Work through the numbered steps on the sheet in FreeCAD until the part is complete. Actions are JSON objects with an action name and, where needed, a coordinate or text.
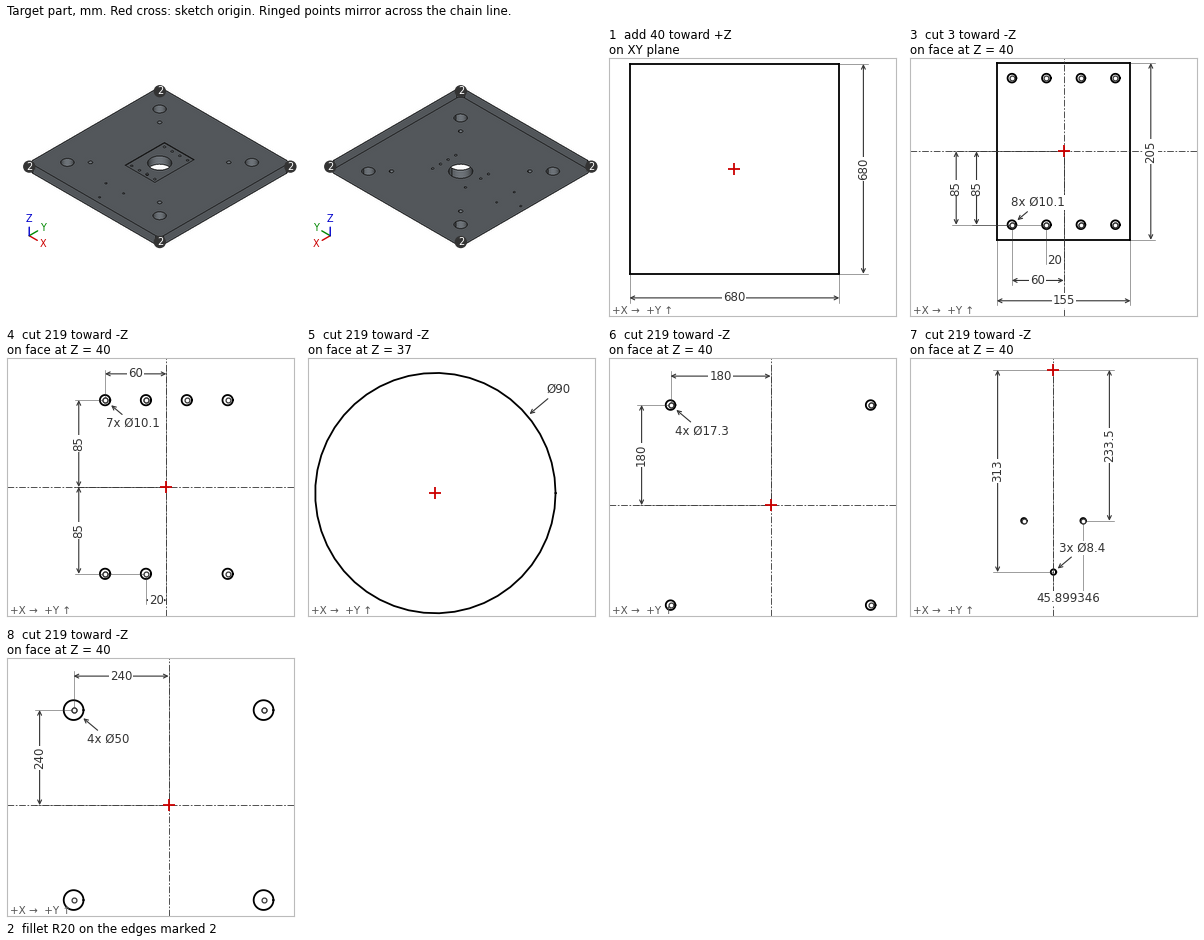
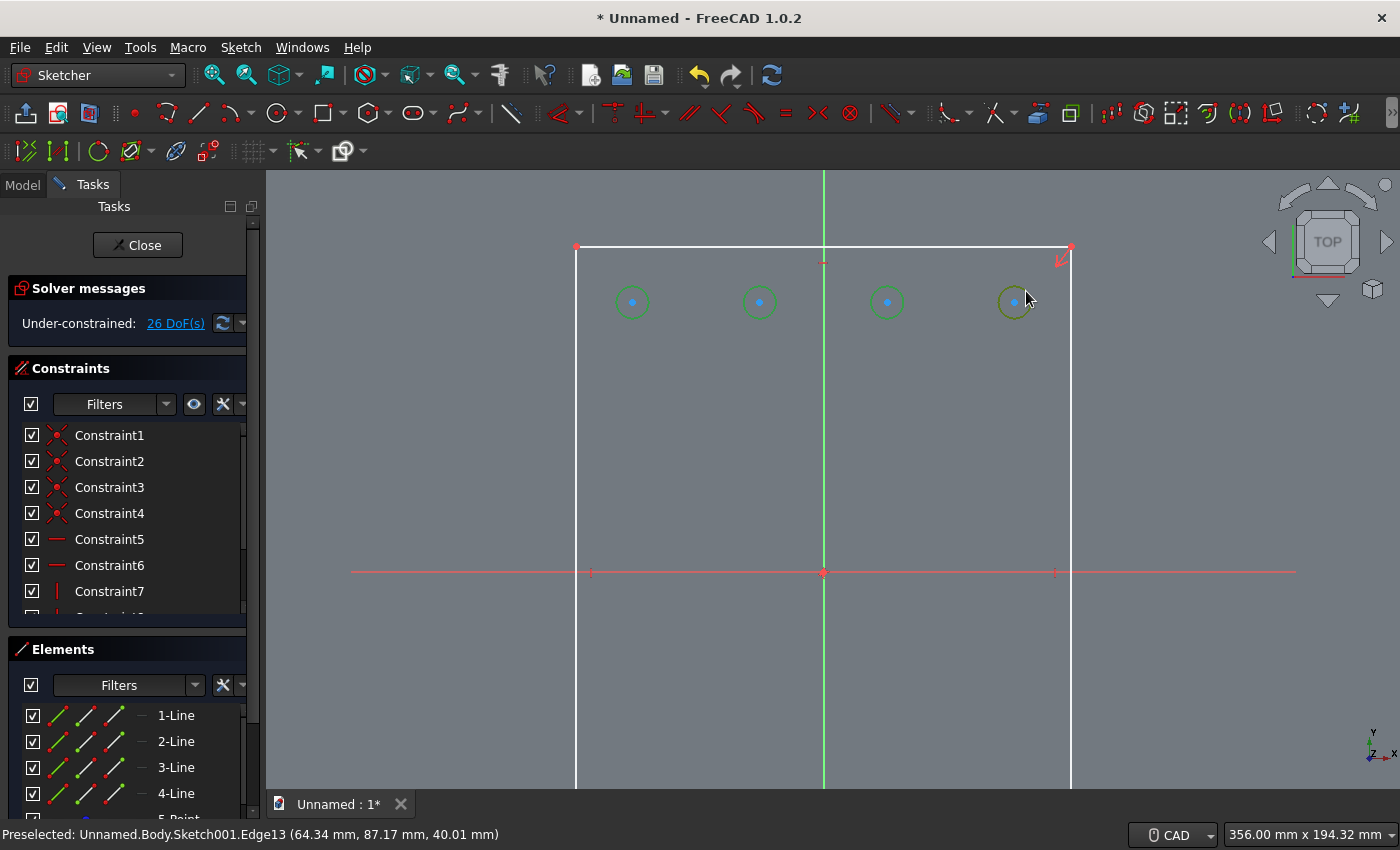
{"action": "left_click", "coordinate": [786, 114]}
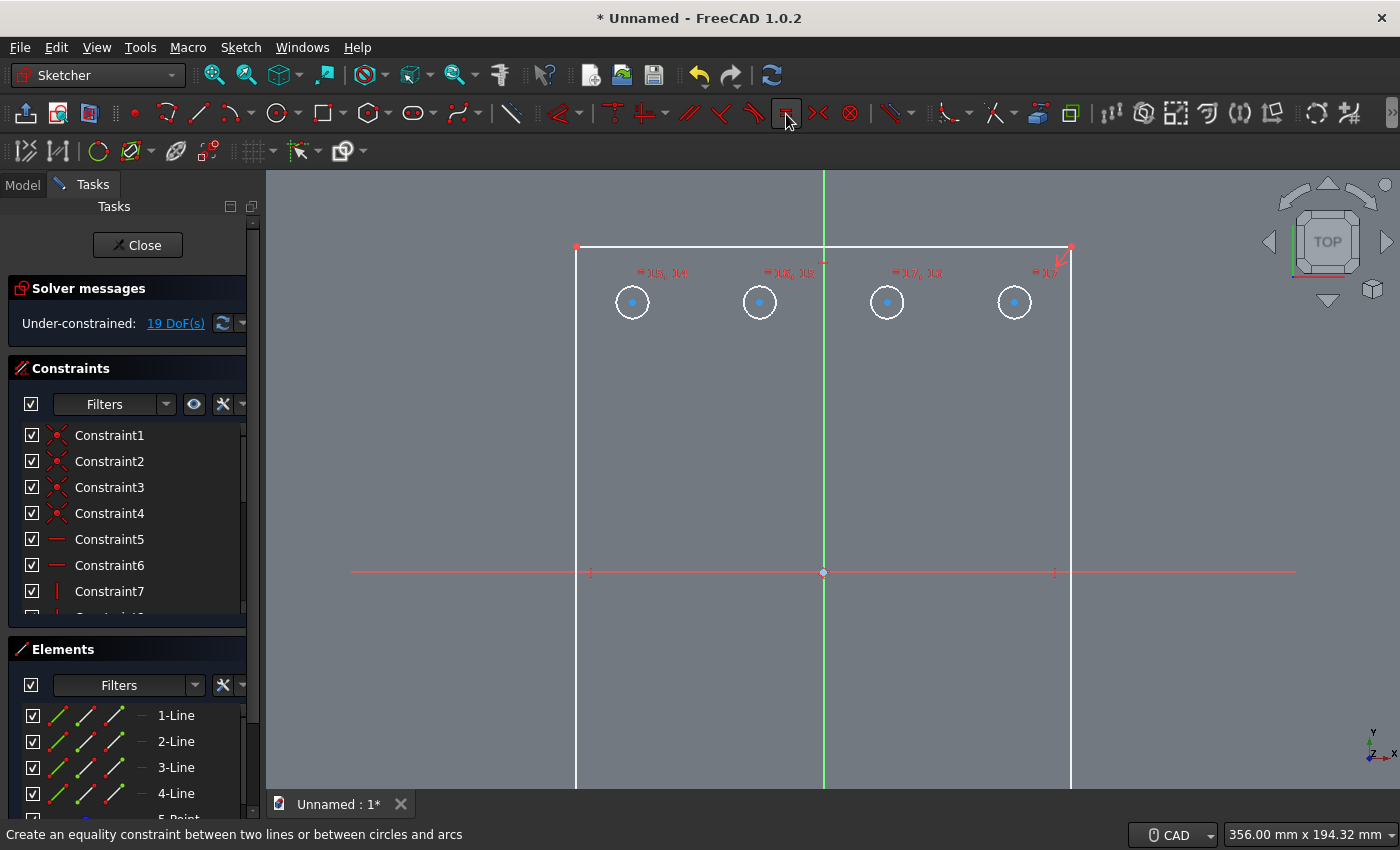
{"action": "scroll", "coordinate": [644, 291], "scroll_direction": "down", "scroll_amount": 2}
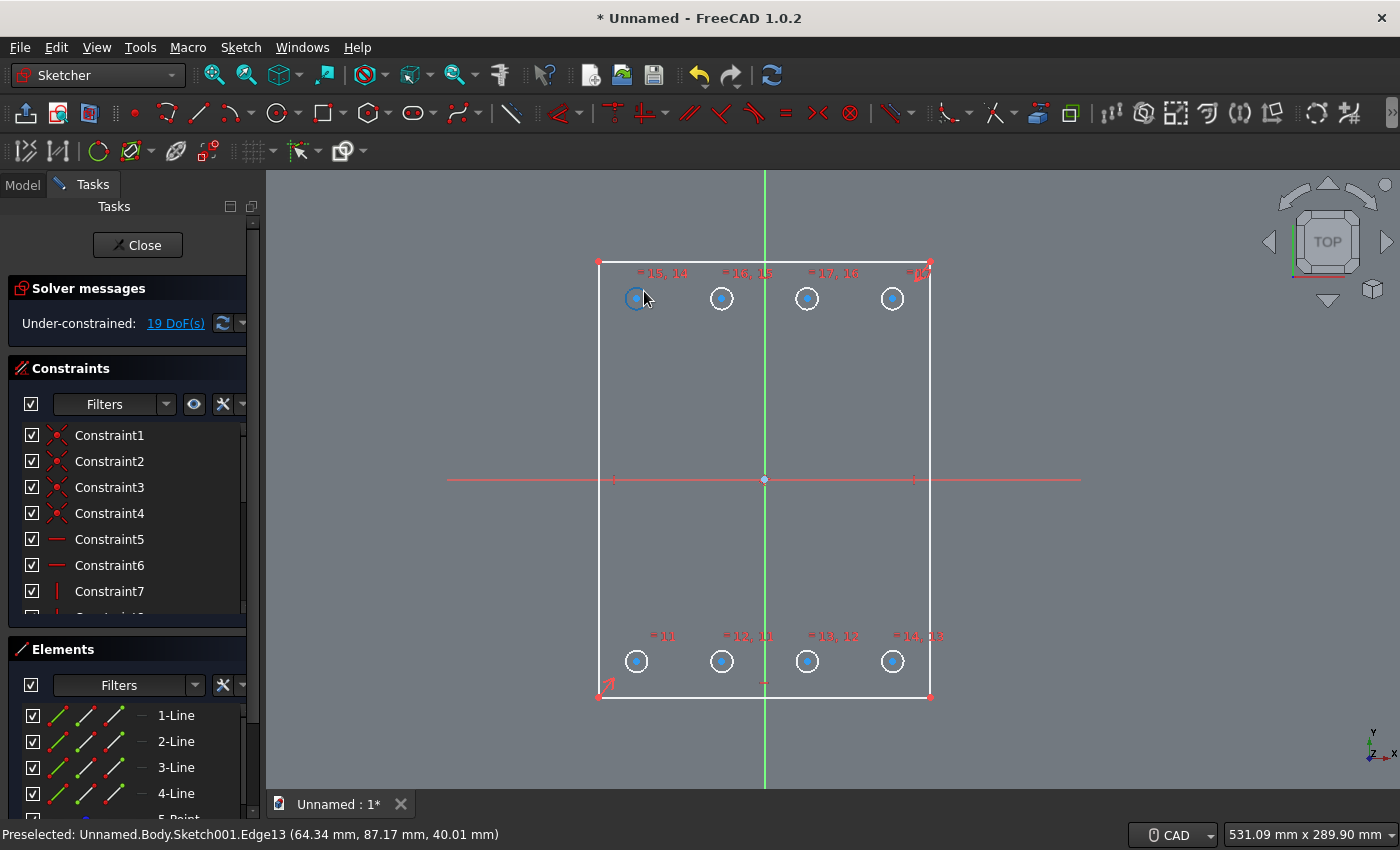
{"action": "left_click", "coordinate": [722, 662]}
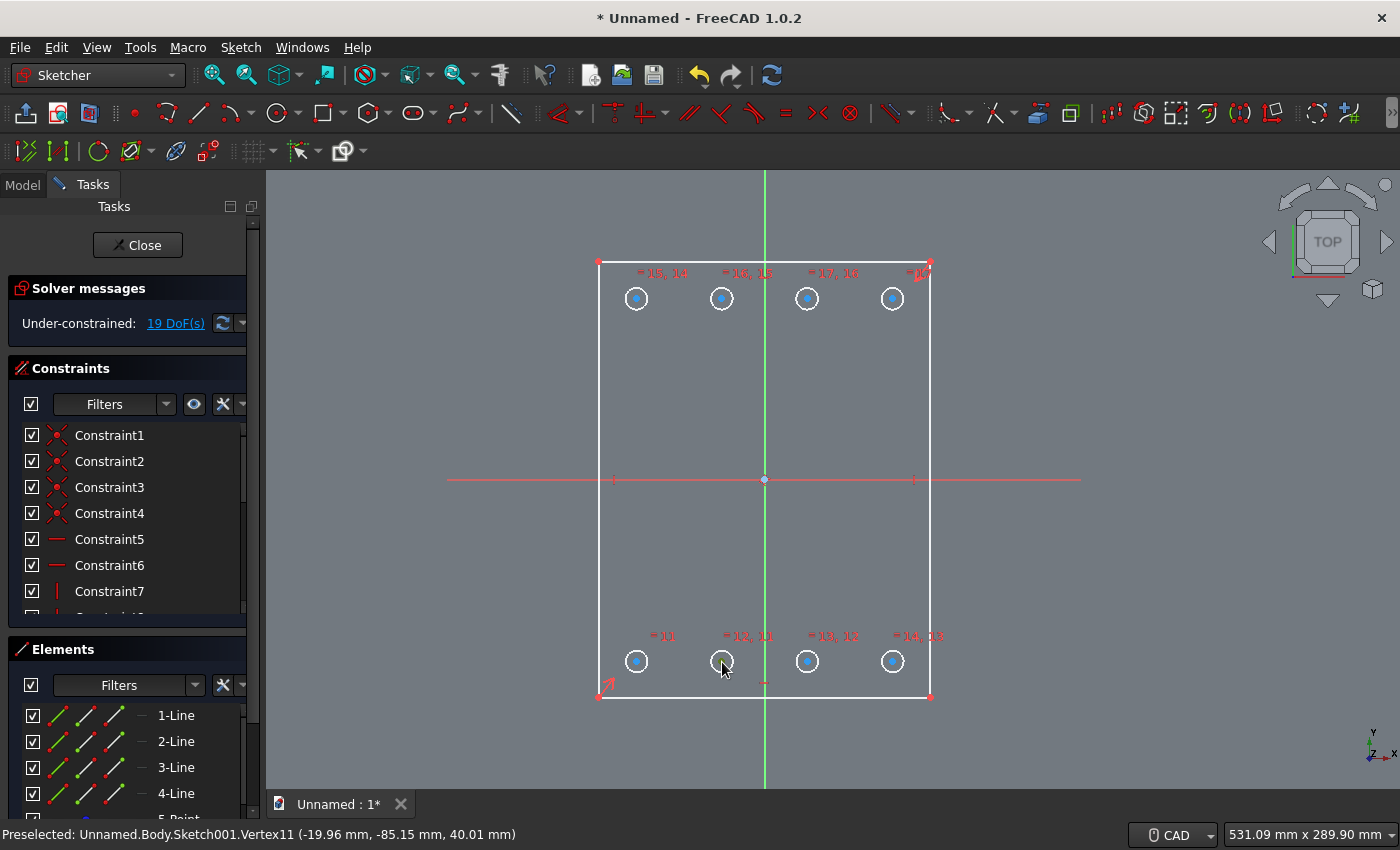
{"action": "left_click", "coordinate": [807, 662]}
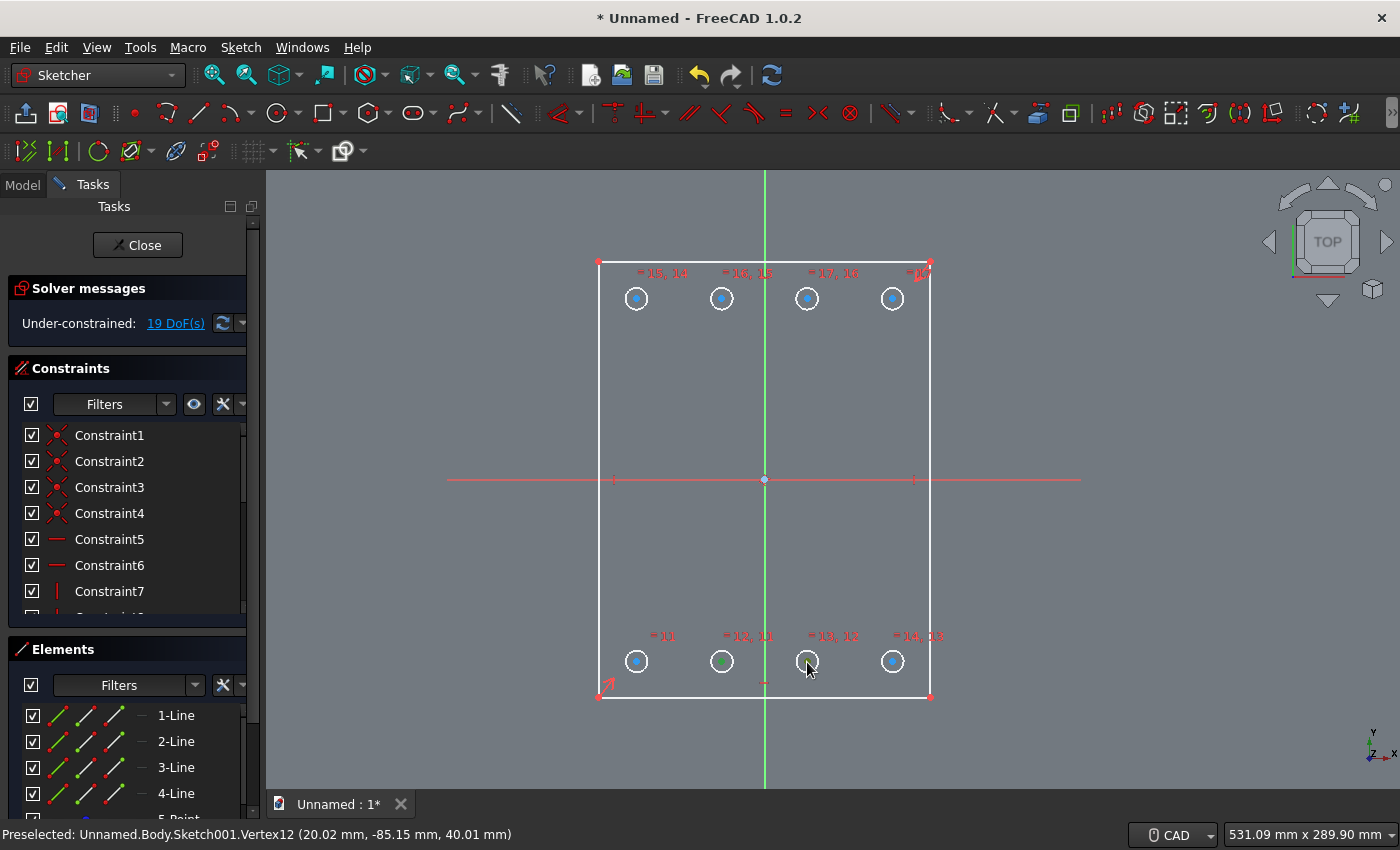
{"action": "left_click", "coordinate": [765, 600]}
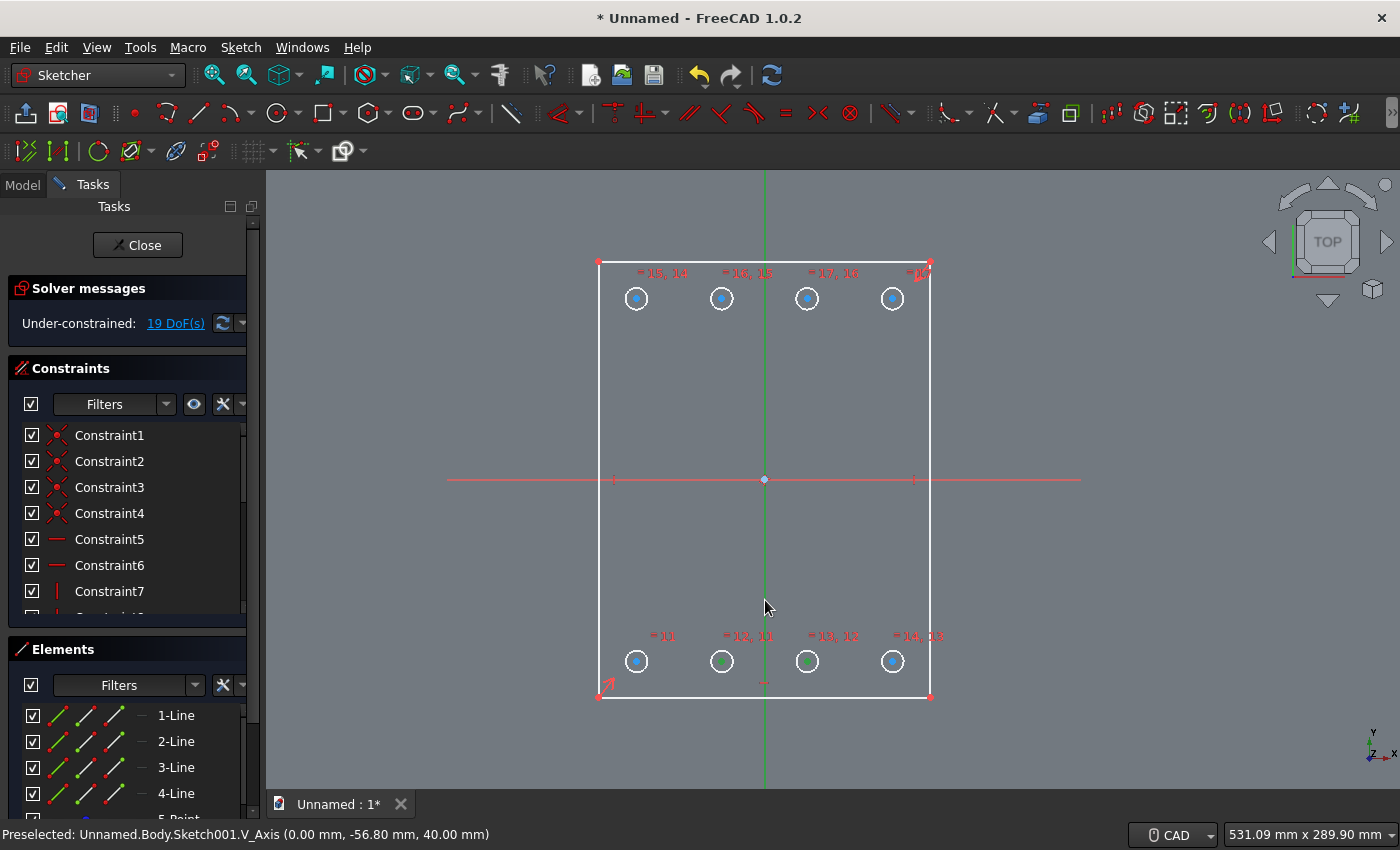
{"action": "left_click", "coordinate": [818, 114]}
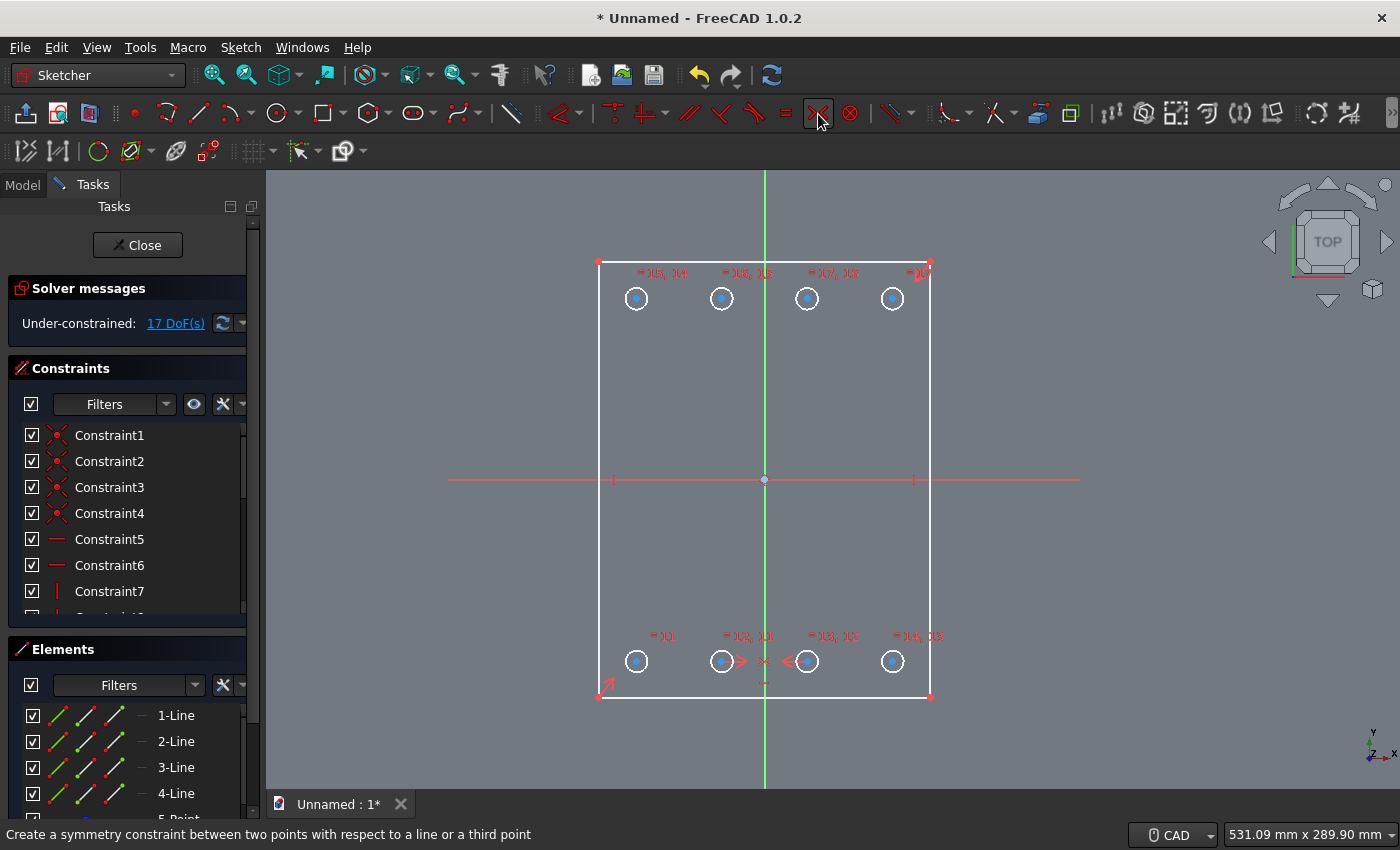
{"action": "left_click", "coordinate": [637, 662]}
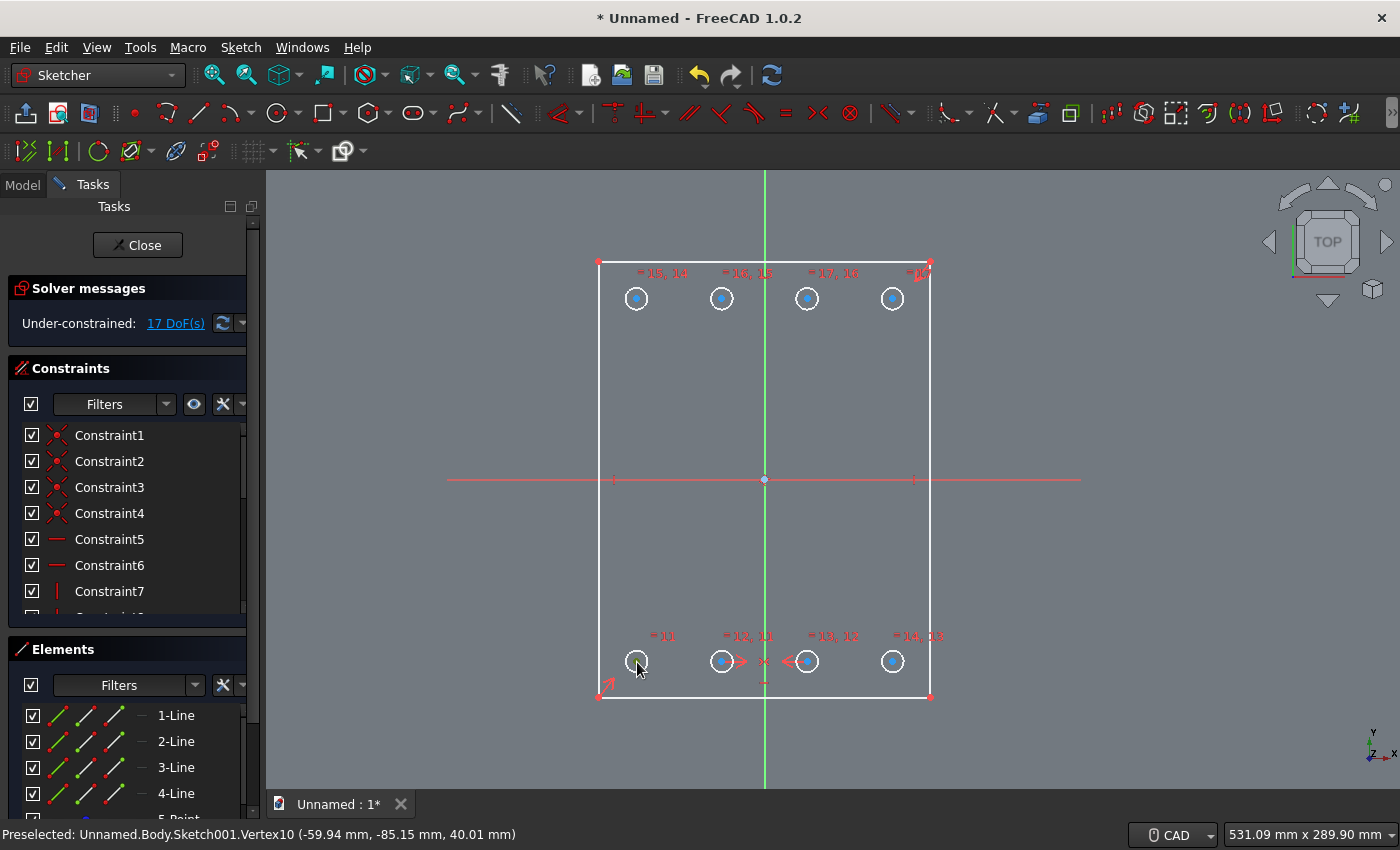
{"action": "left_click", "coordinate": [893, 662]}